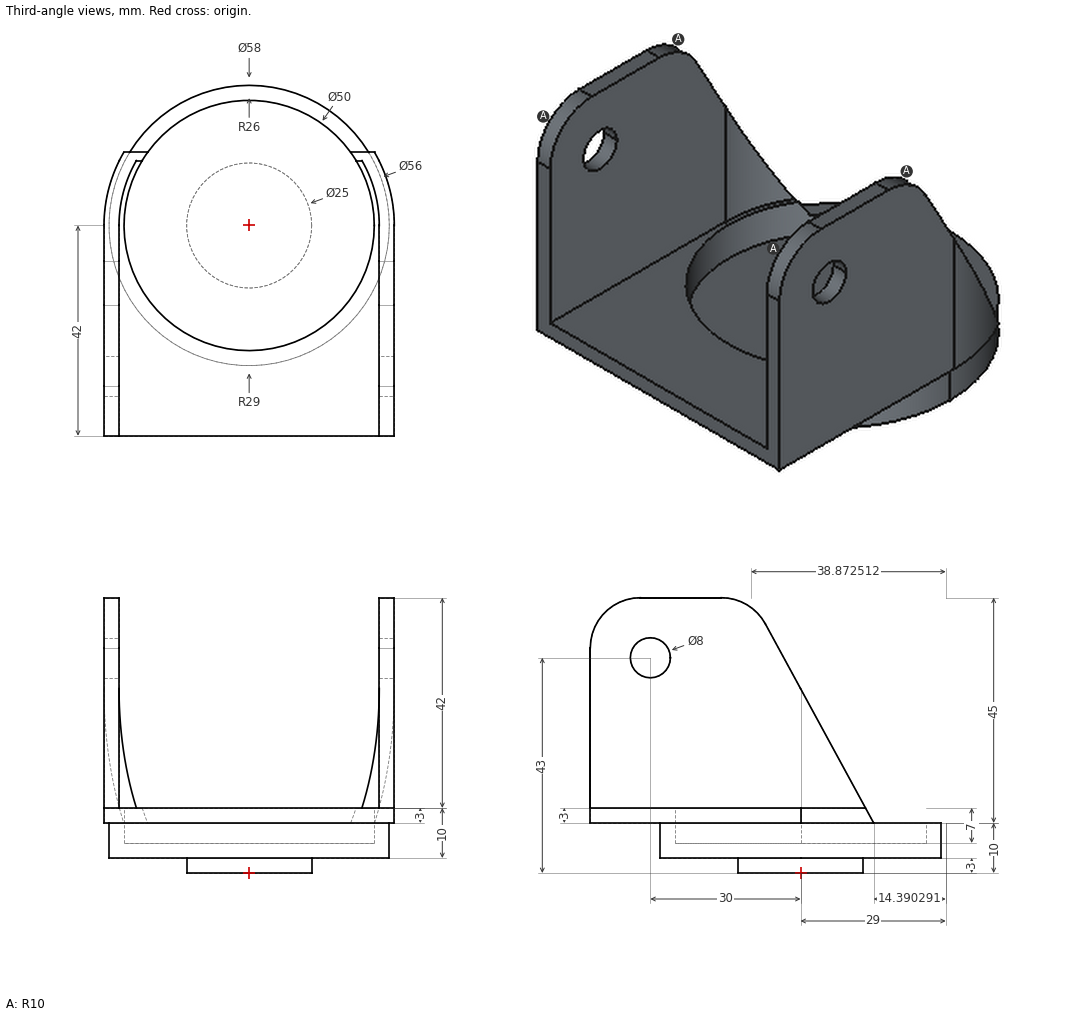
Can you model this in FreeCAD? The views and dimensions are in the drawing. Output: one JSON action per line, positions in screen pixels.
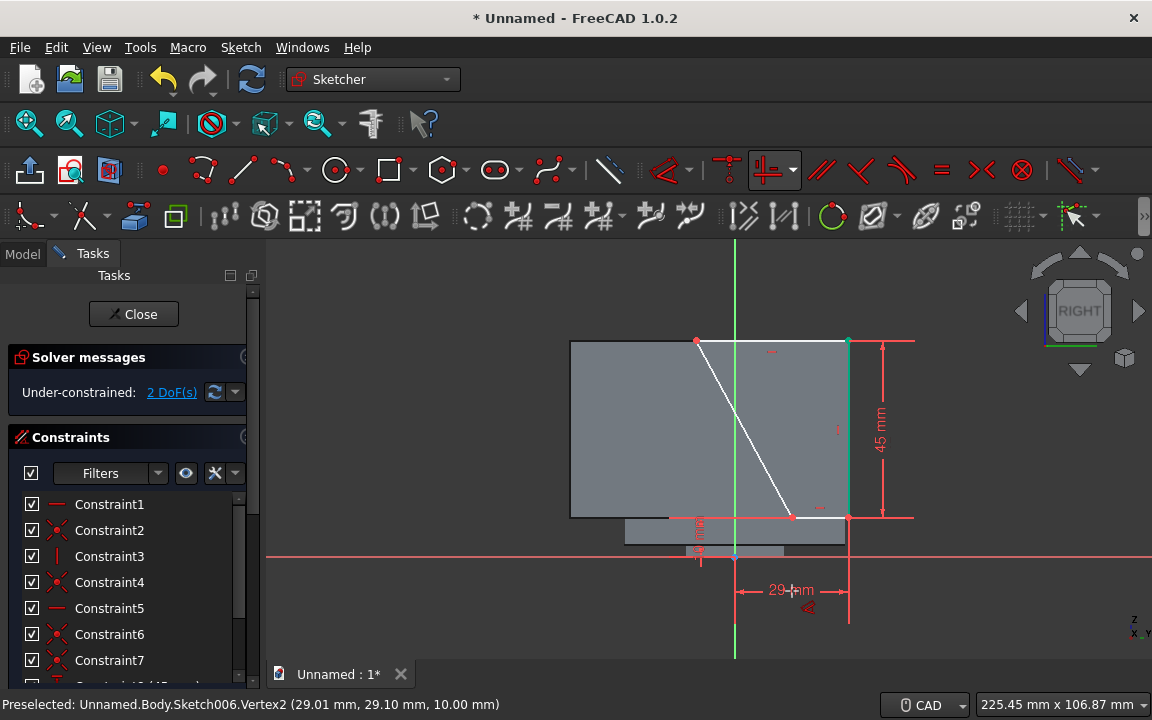
{"action": "left_click", "coordinate": [809, 518]}
{"action": "left_click", "coordinate": [820, 484]}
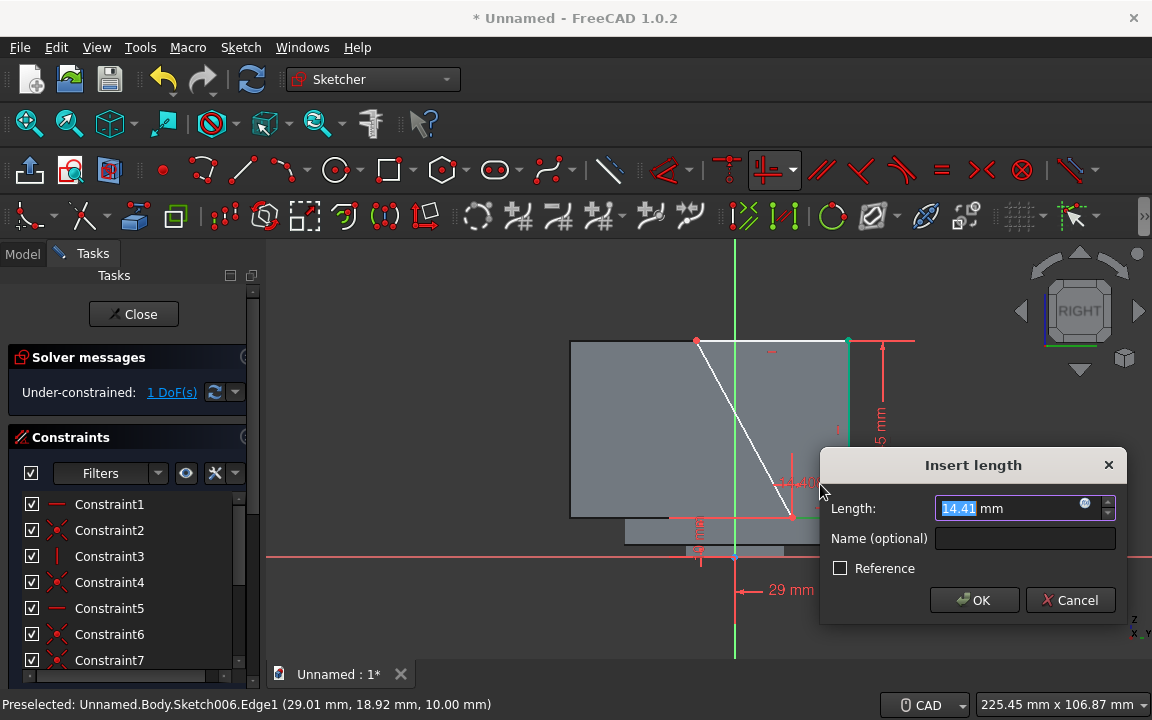
{"action": "type", "text": "14.390291"}
{"action": "key", "text": "Return"}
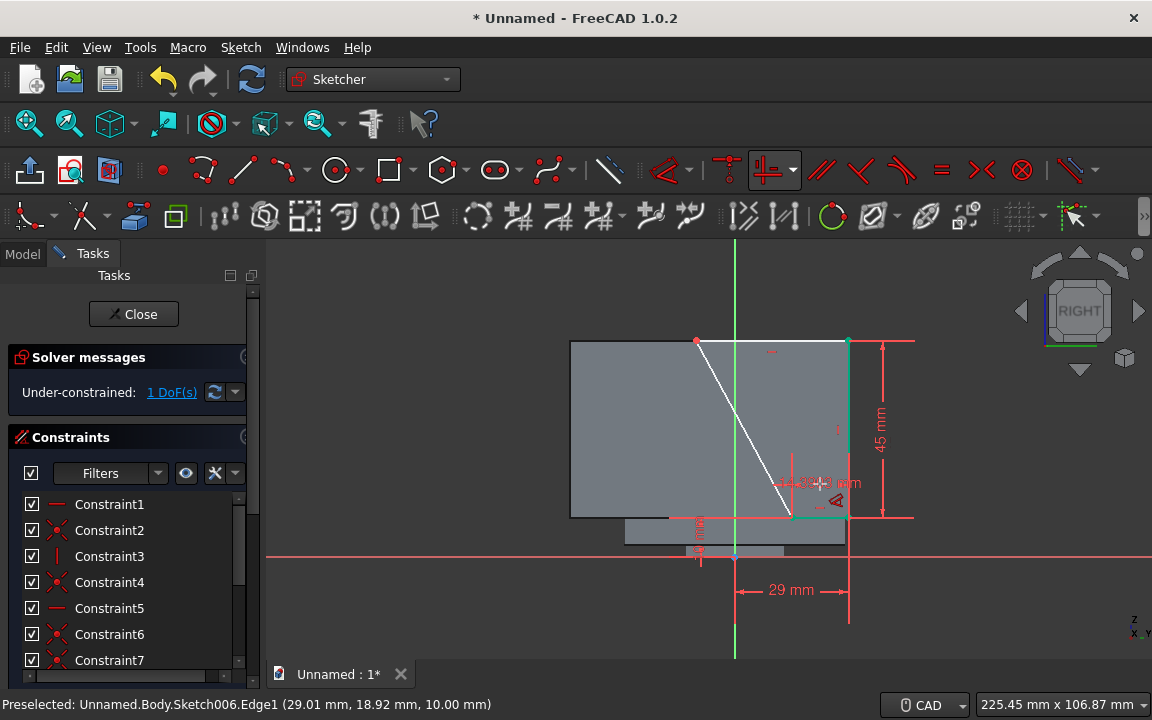
{"action": "left_click", "coordinate": [803, 341]}
{"action": "left_click", "coordinate": [772, 307]}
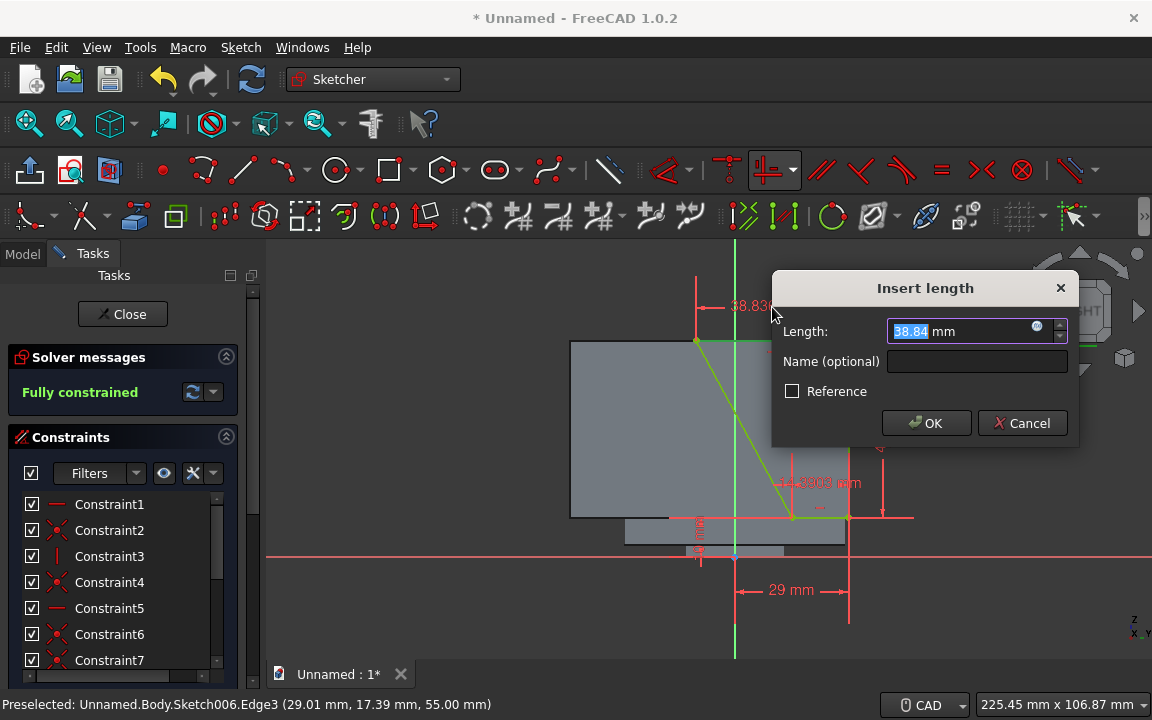
{"action": "type", "text": "38.872512"}
{"action": "key", "text": "Return"}
{"action": "key", "text": "Escape"}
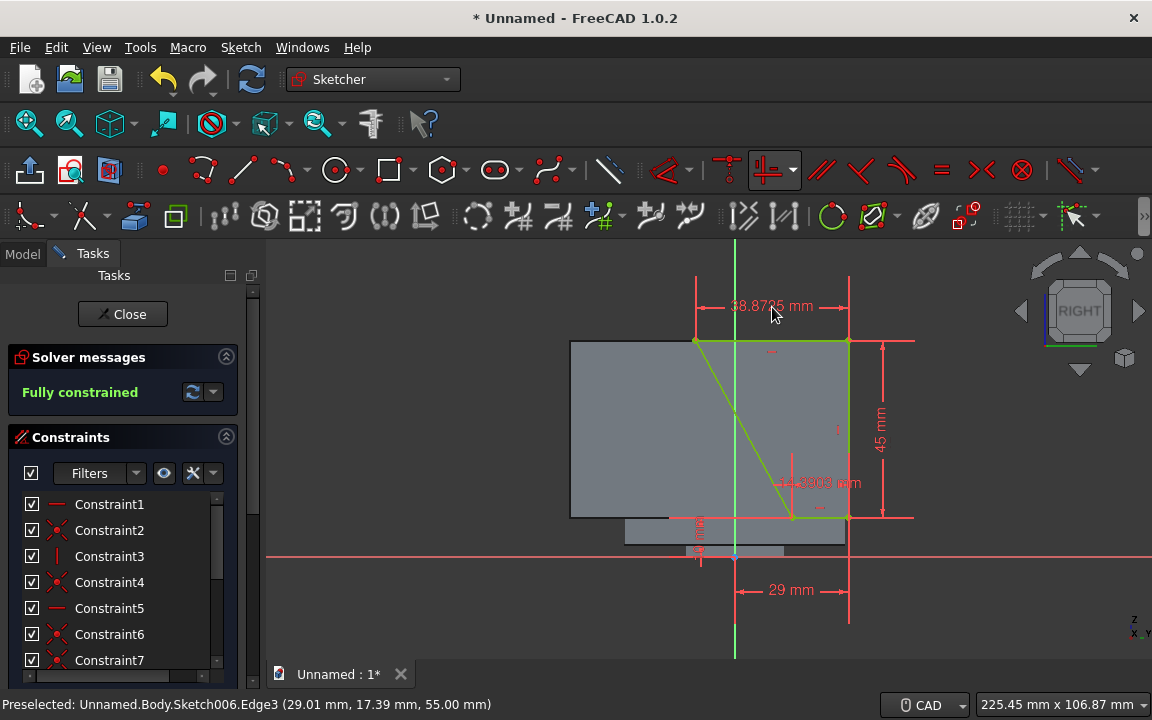
{"action": "left_click", "coordinate": [123, 314]}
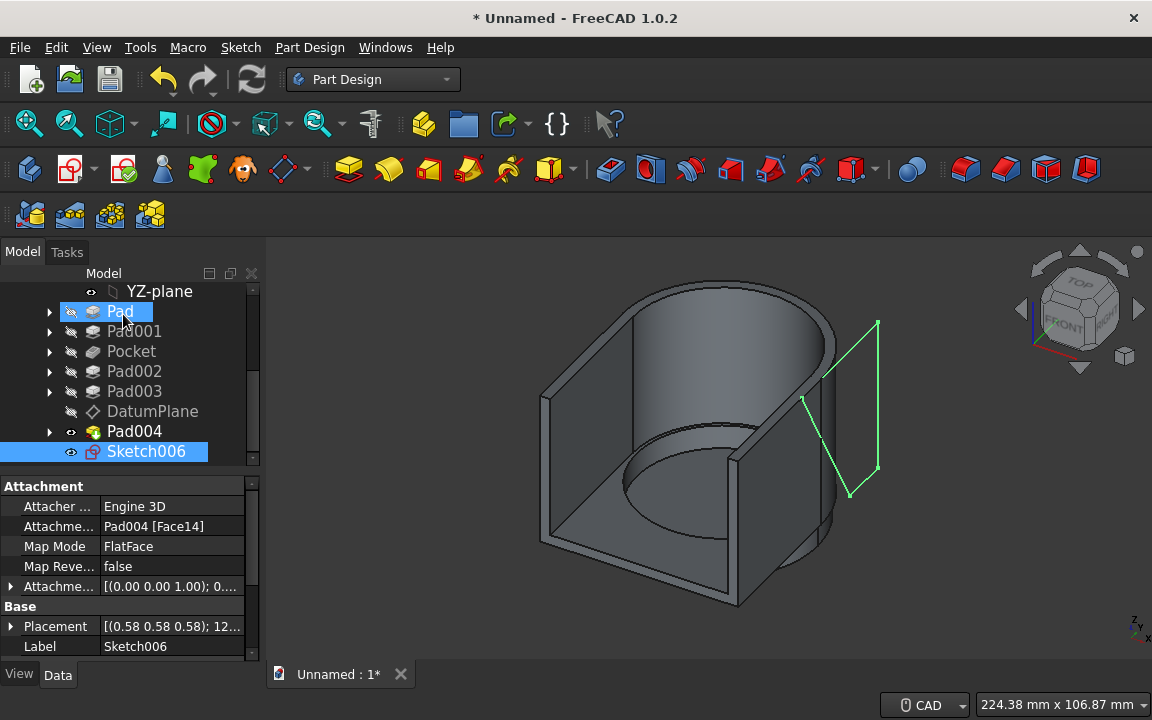
{"action": "left_click", "coordinate": [612, 170]}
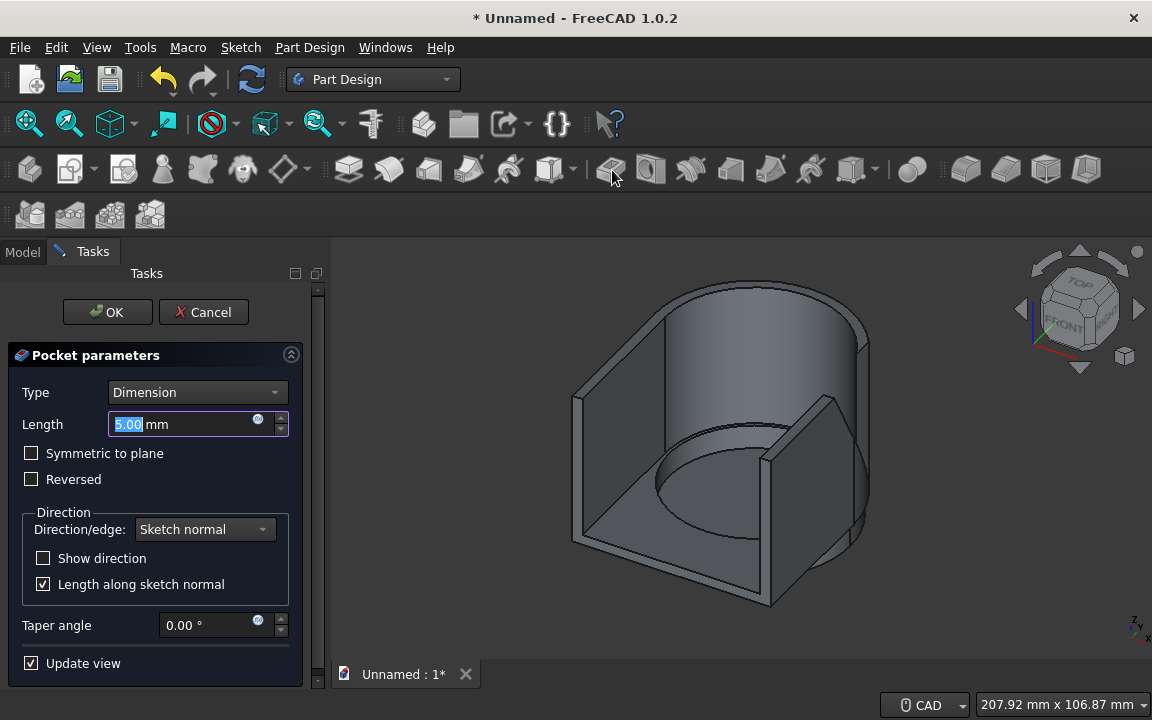
{"action": "left_click", "coordinate": [198, 392]}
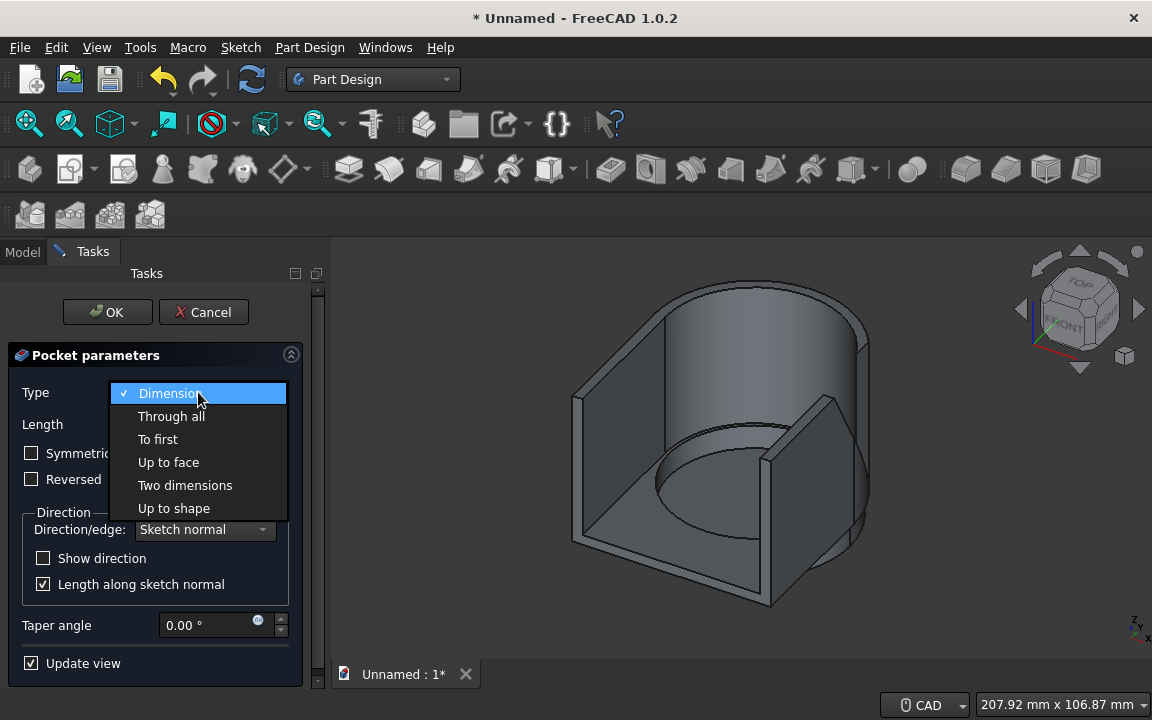
{"action": "left_click", "coordinate": [198, 416]}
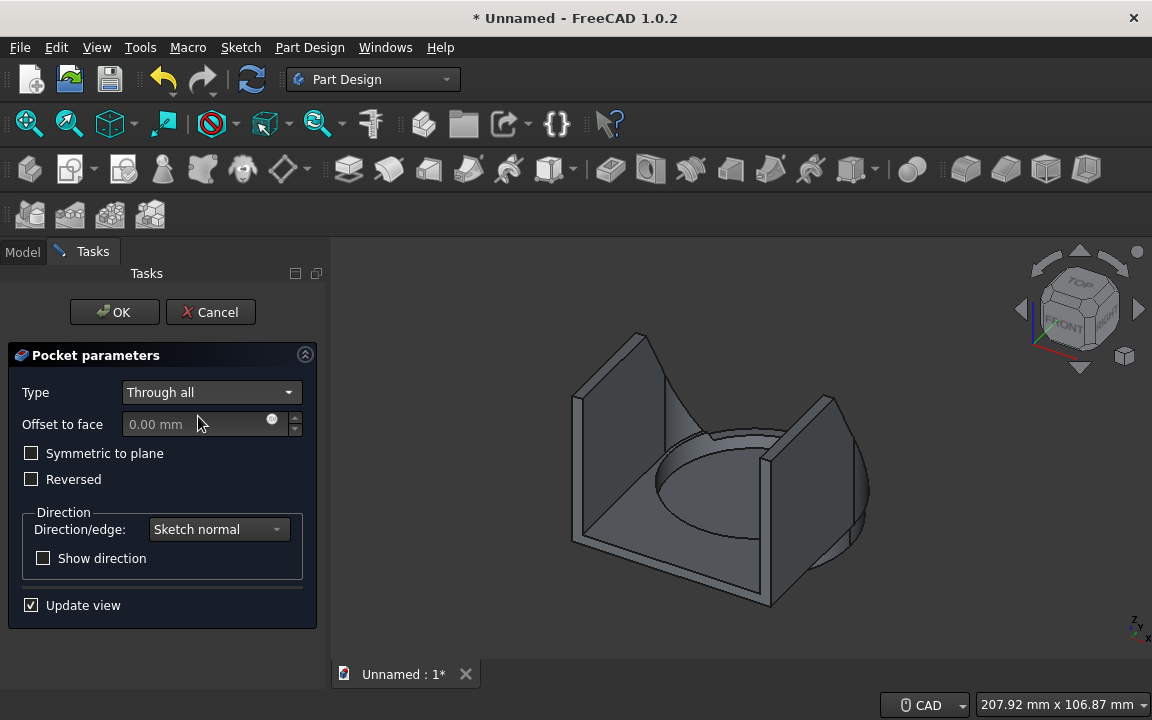
{"action": "left_click", "coordinate": [115, 312]}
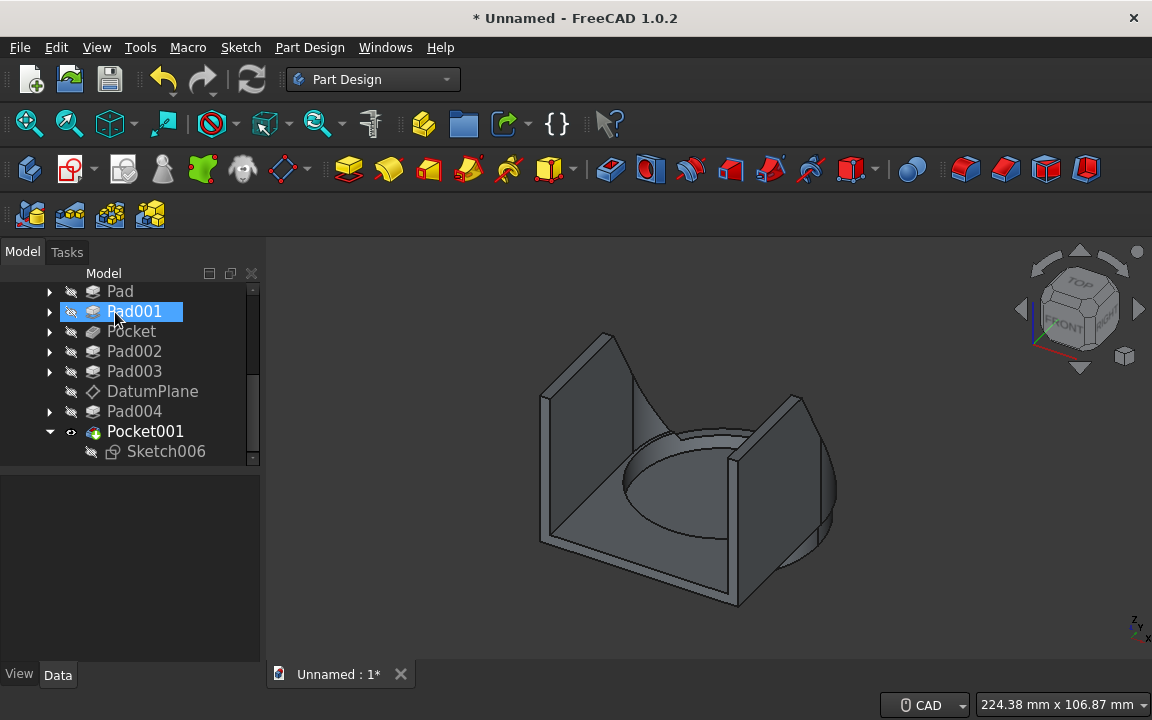
{"action": "left_click", "coordinate": [732, 458]}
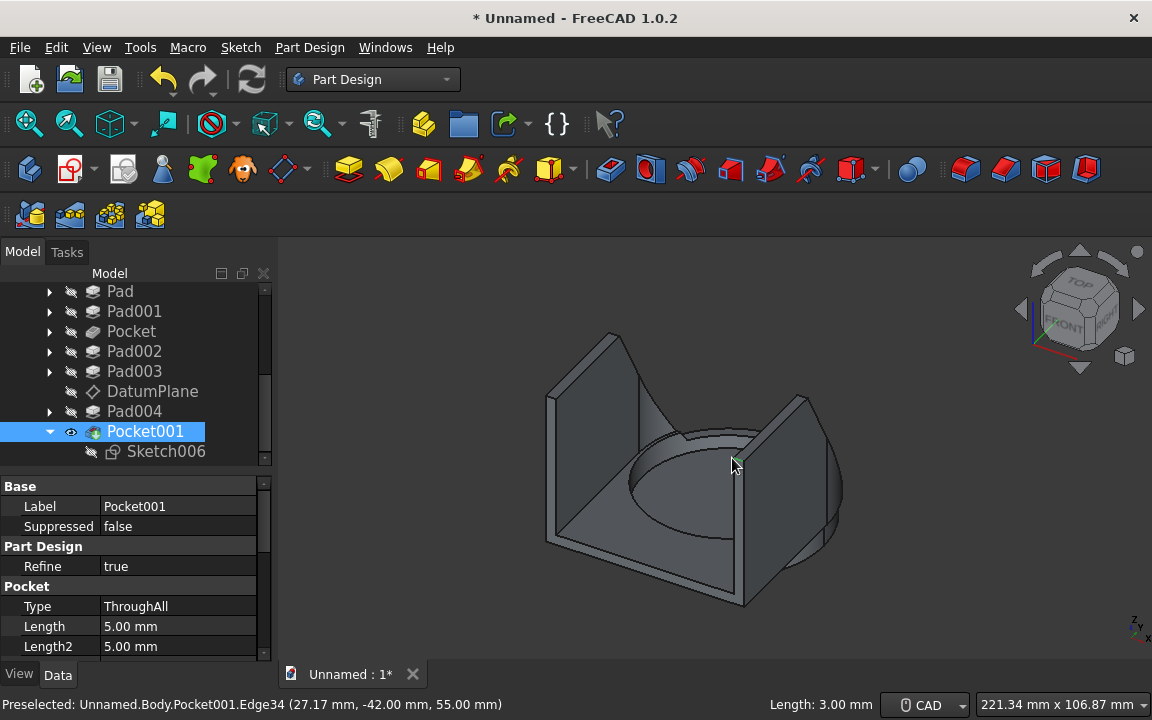
{"action": "left_click", "coordinate": [550, 396], "text": "ctrl"}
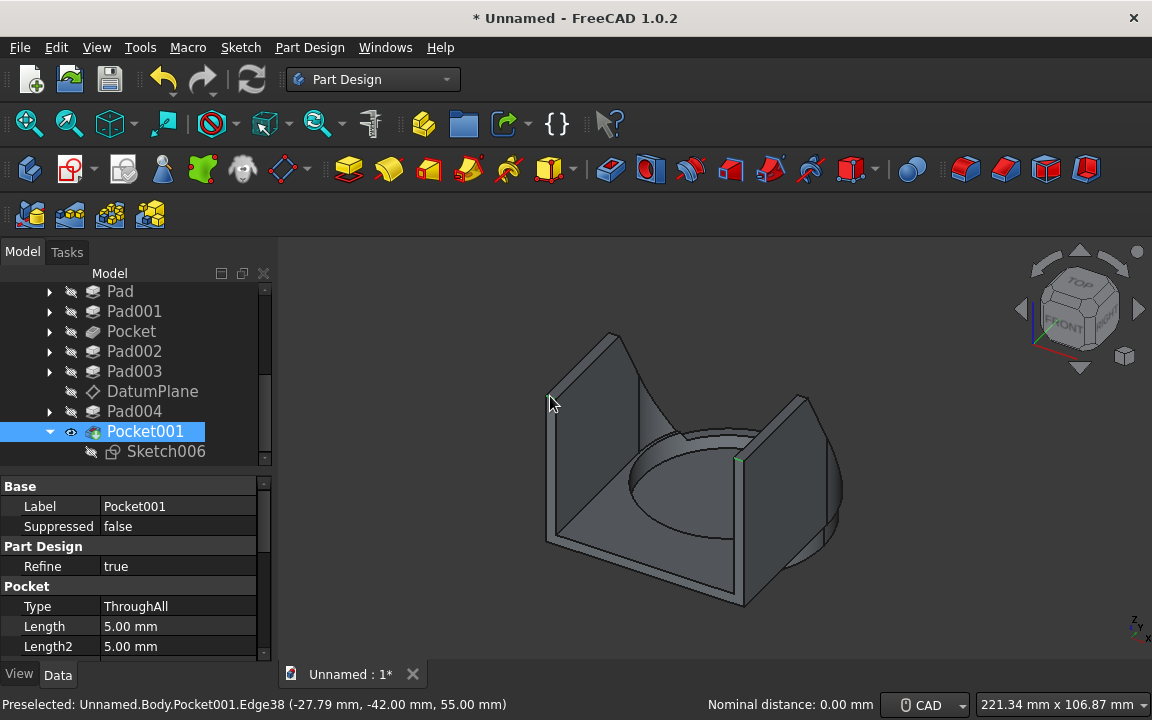
{"action": "scroll", "coordinate": [802, 396], "scroll_direction": "up", "scroll_amount": 7}